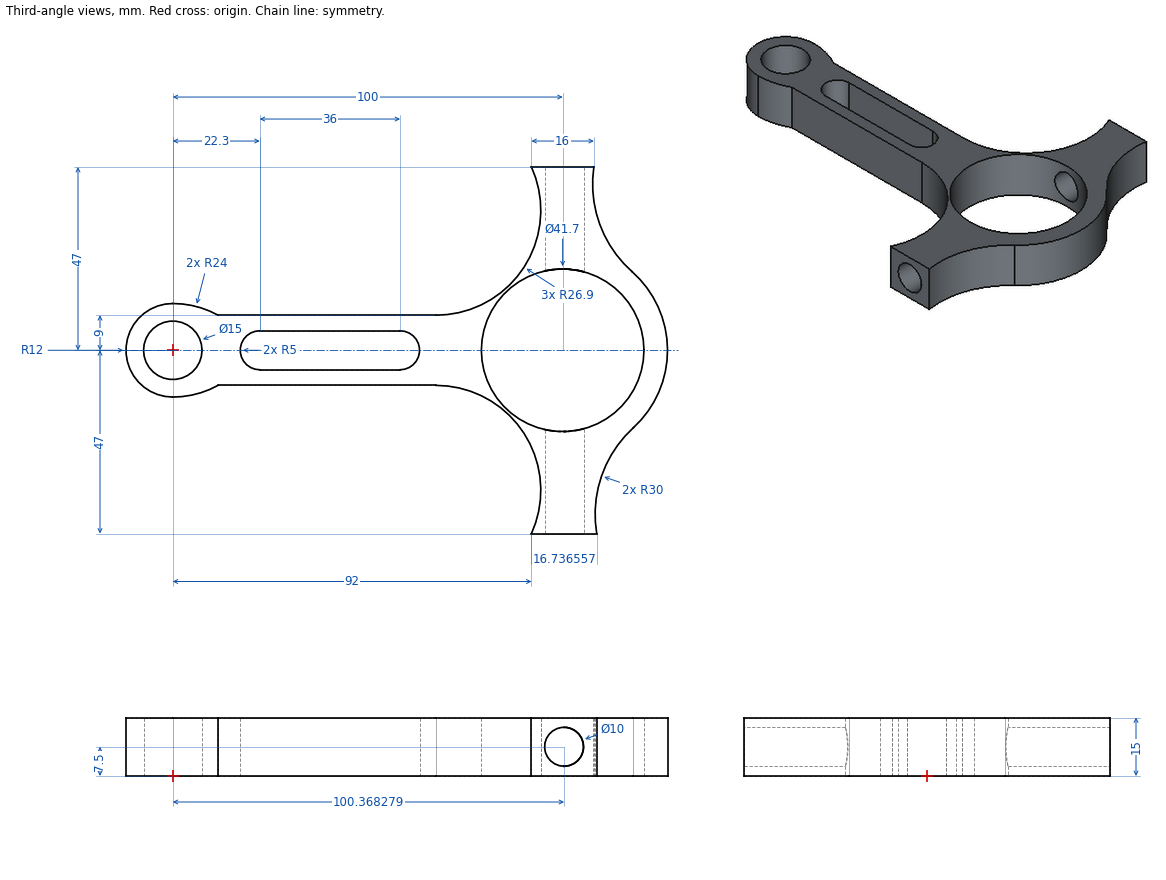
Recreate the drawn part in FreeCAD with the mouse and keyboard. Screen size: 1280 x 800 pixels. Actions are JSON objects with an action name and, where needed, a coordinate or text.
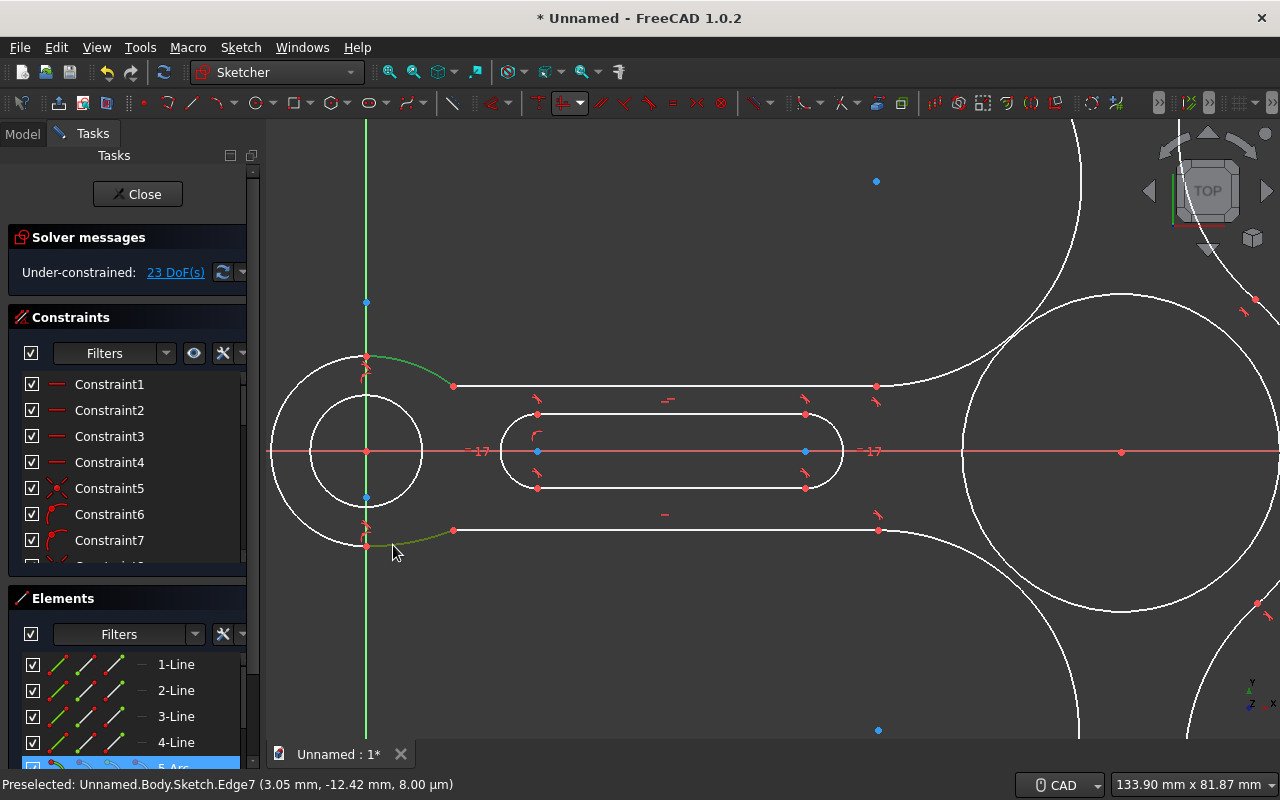
{"action": "left_click", "coordinate": [674, 104]}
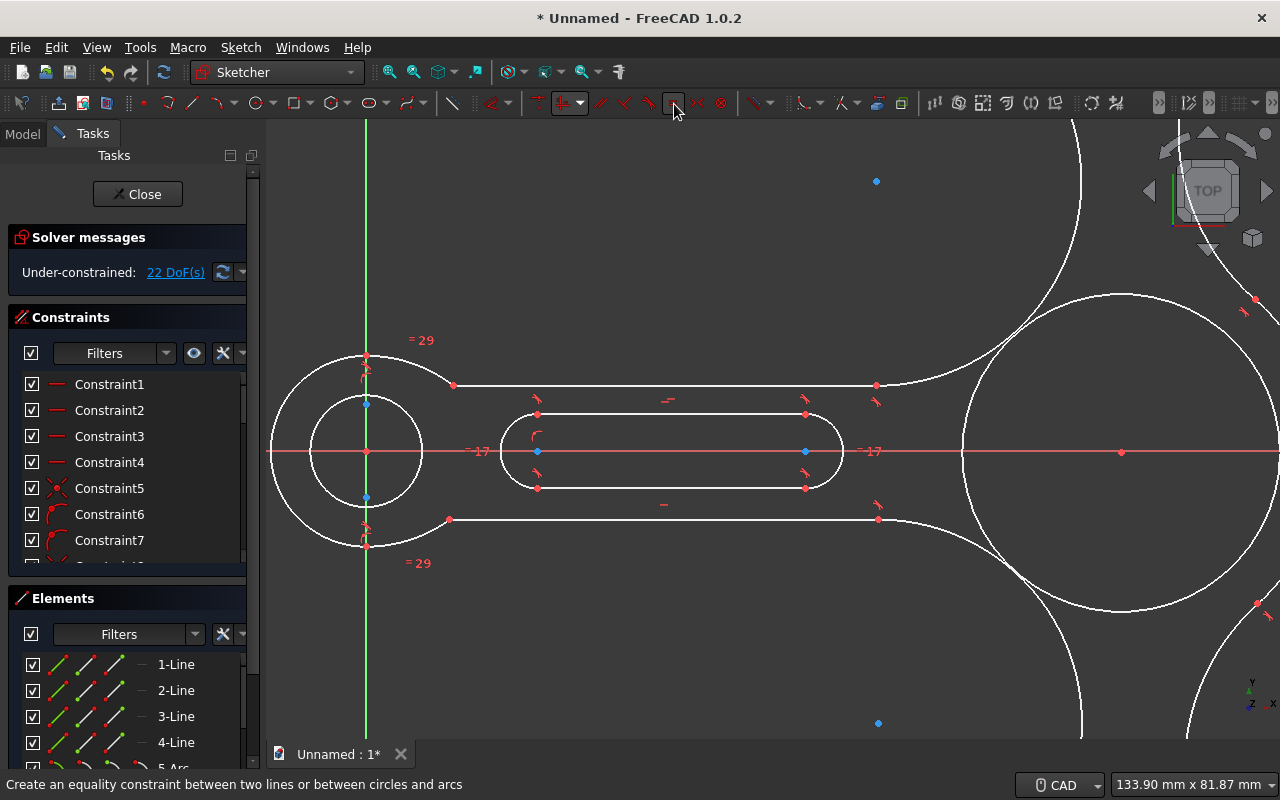
{"action": "left_click", "coordinate": [1079, 689]}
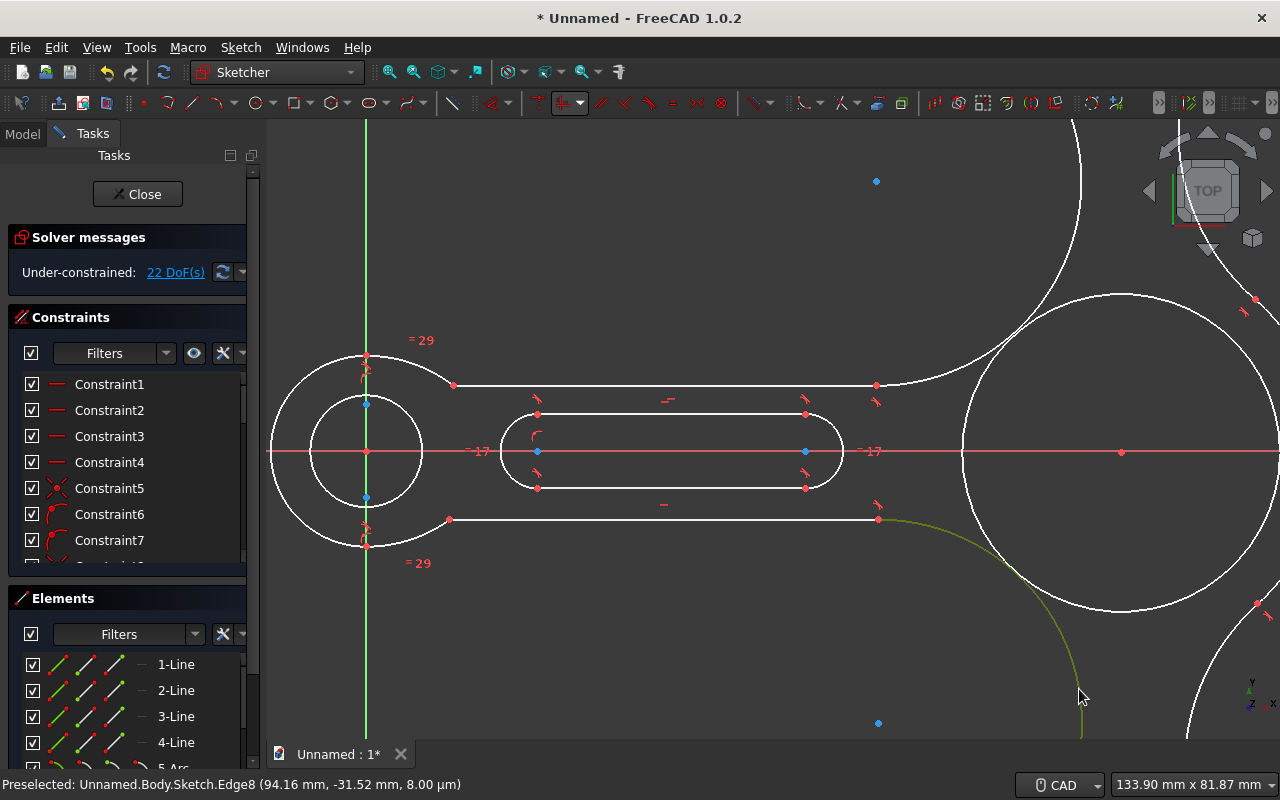
{"action": "scroll", "coordinate": [587, 402], "scroll_direction": "down", "scroll_amount": 3}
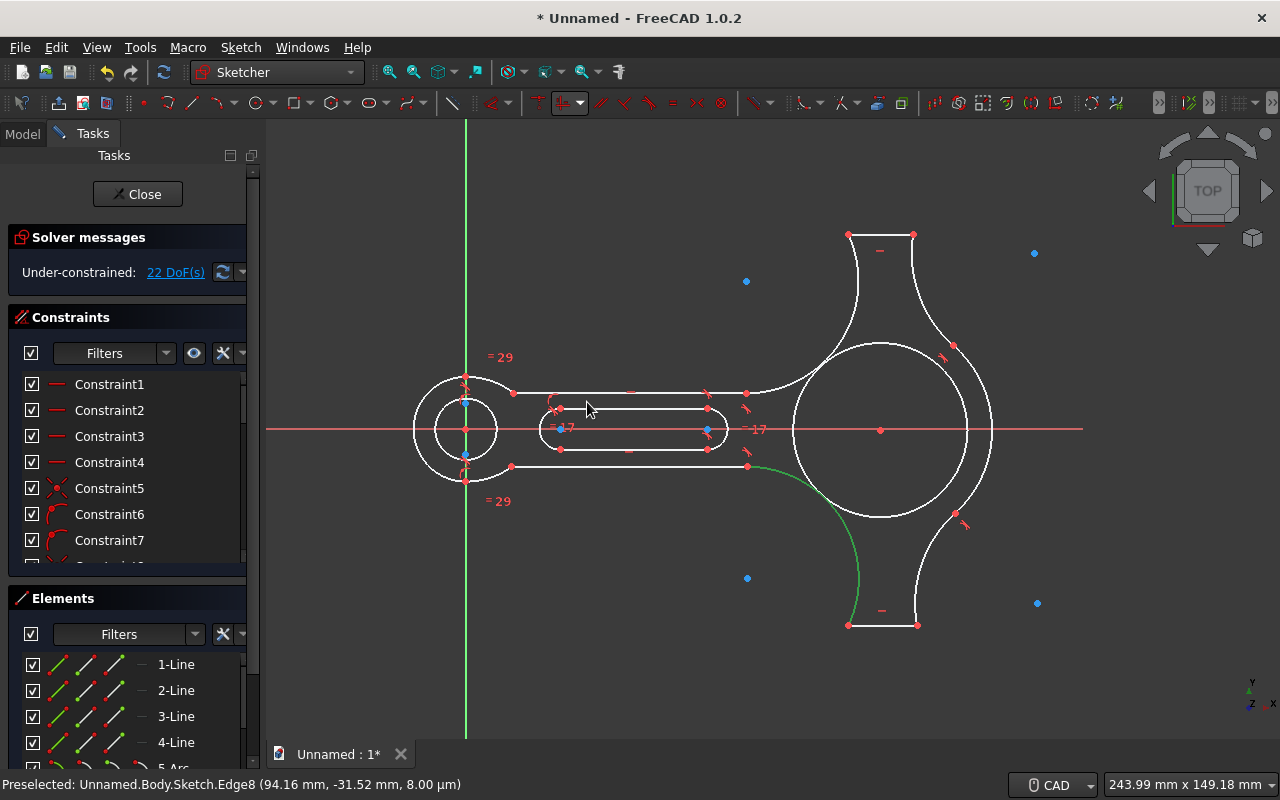
{"action": "left_click", "coordinate": [986, 466]}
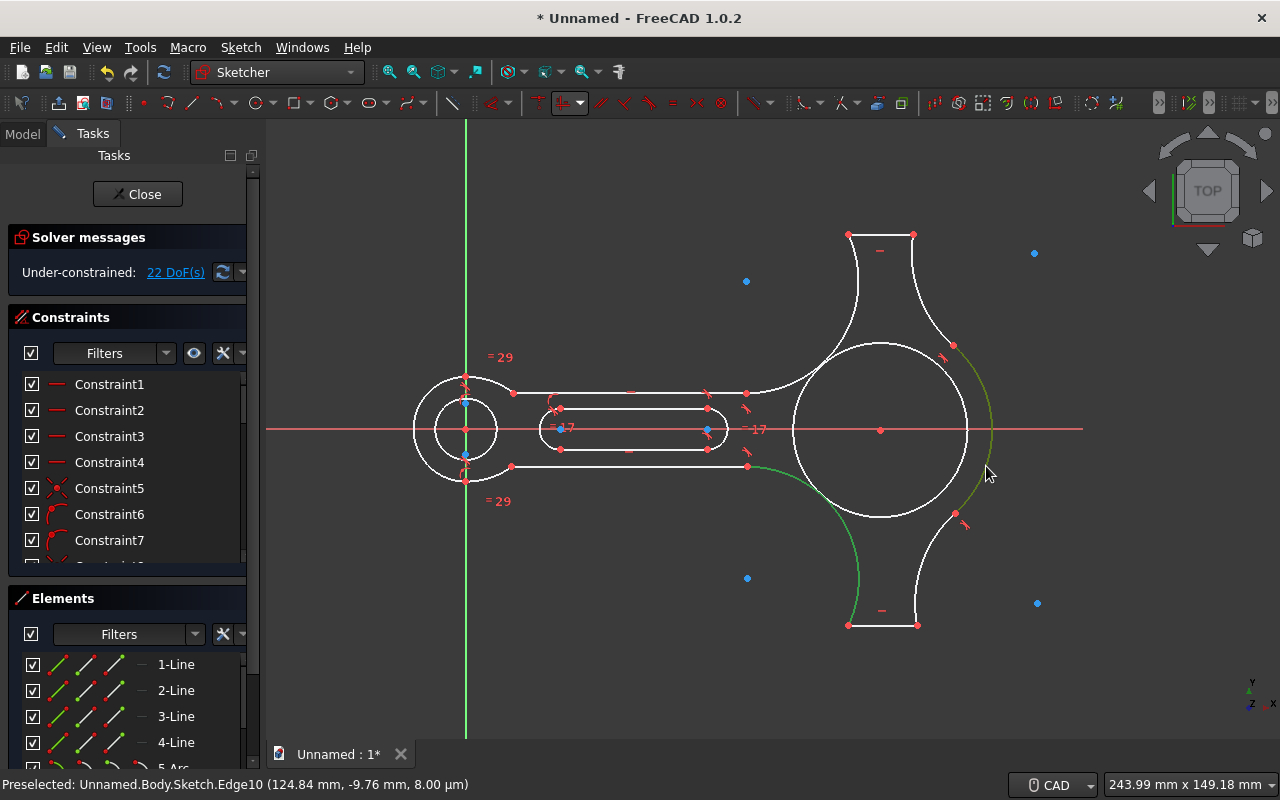
{"action": "left_click", "coordinate": [857, 300]}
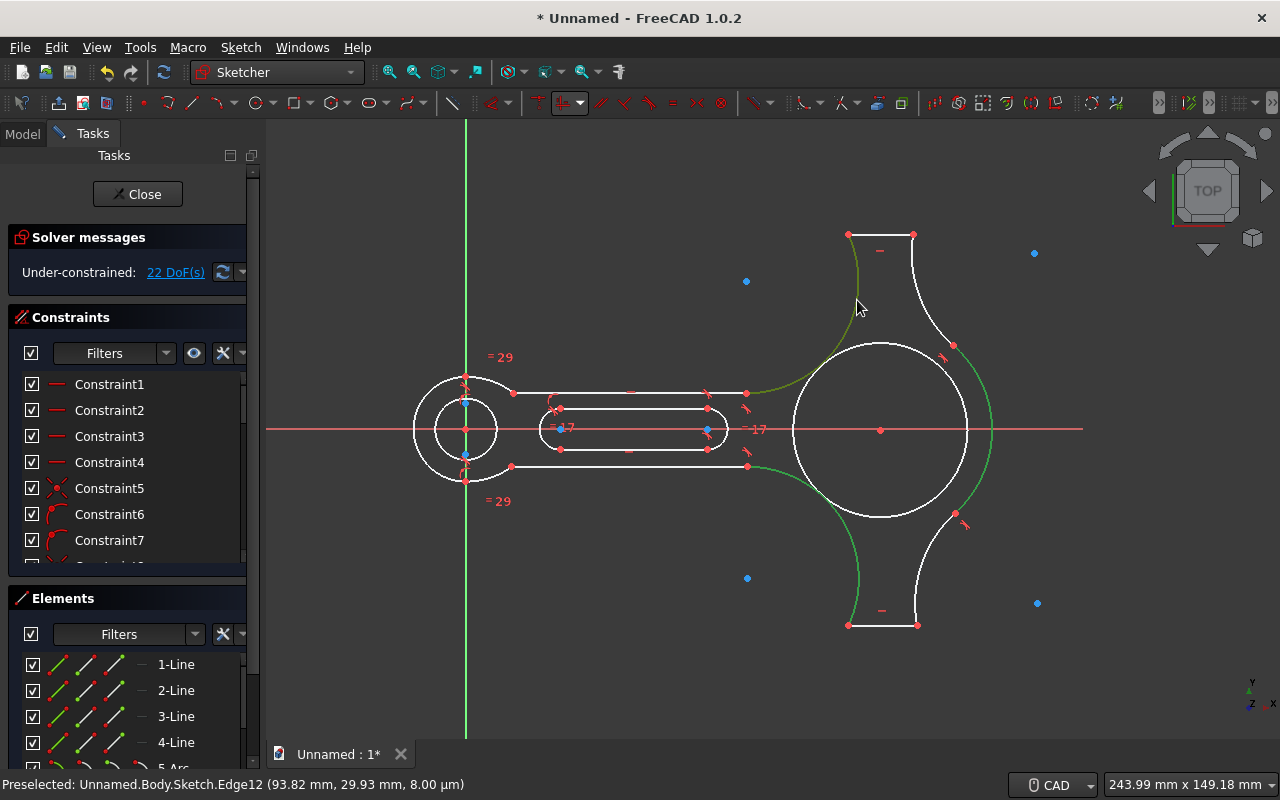
{"action": "left_click", "coordinate": [674, 104]}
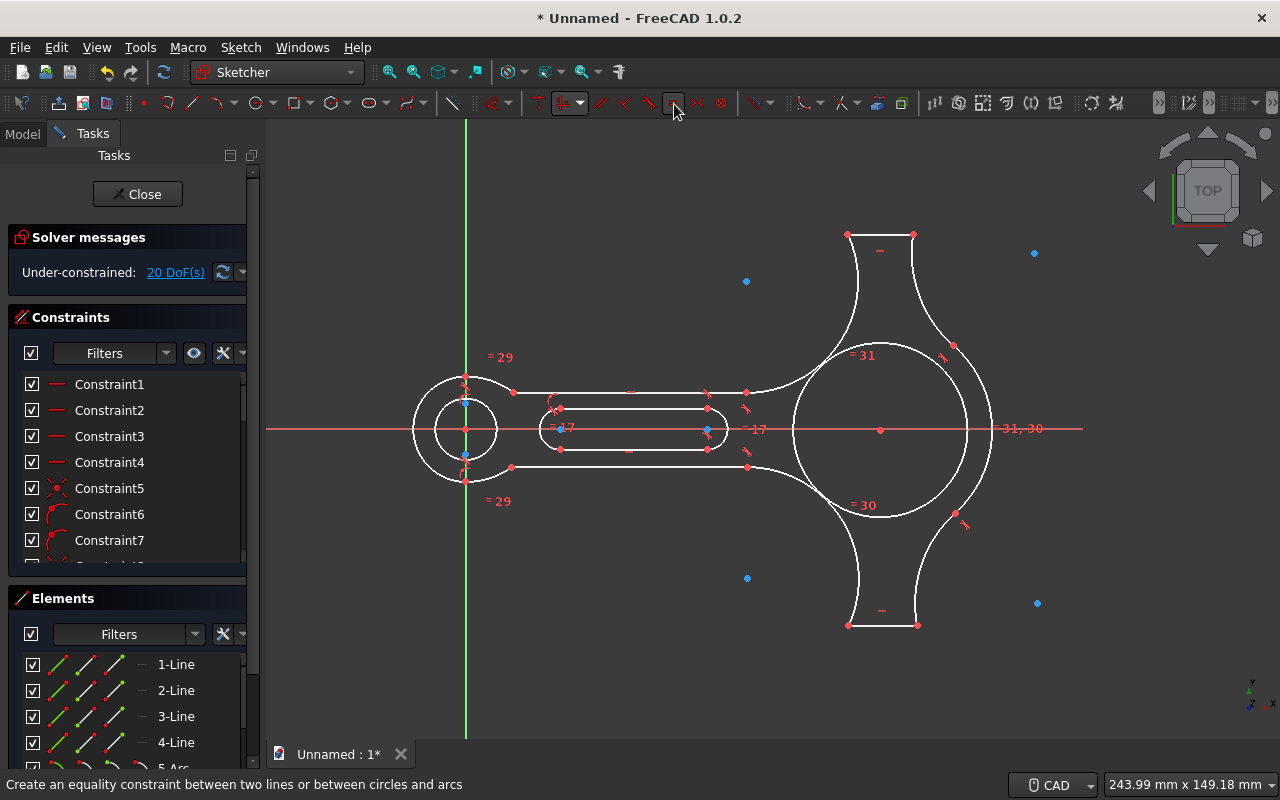
{"action": "left_click", "coordinate": [932, 542]}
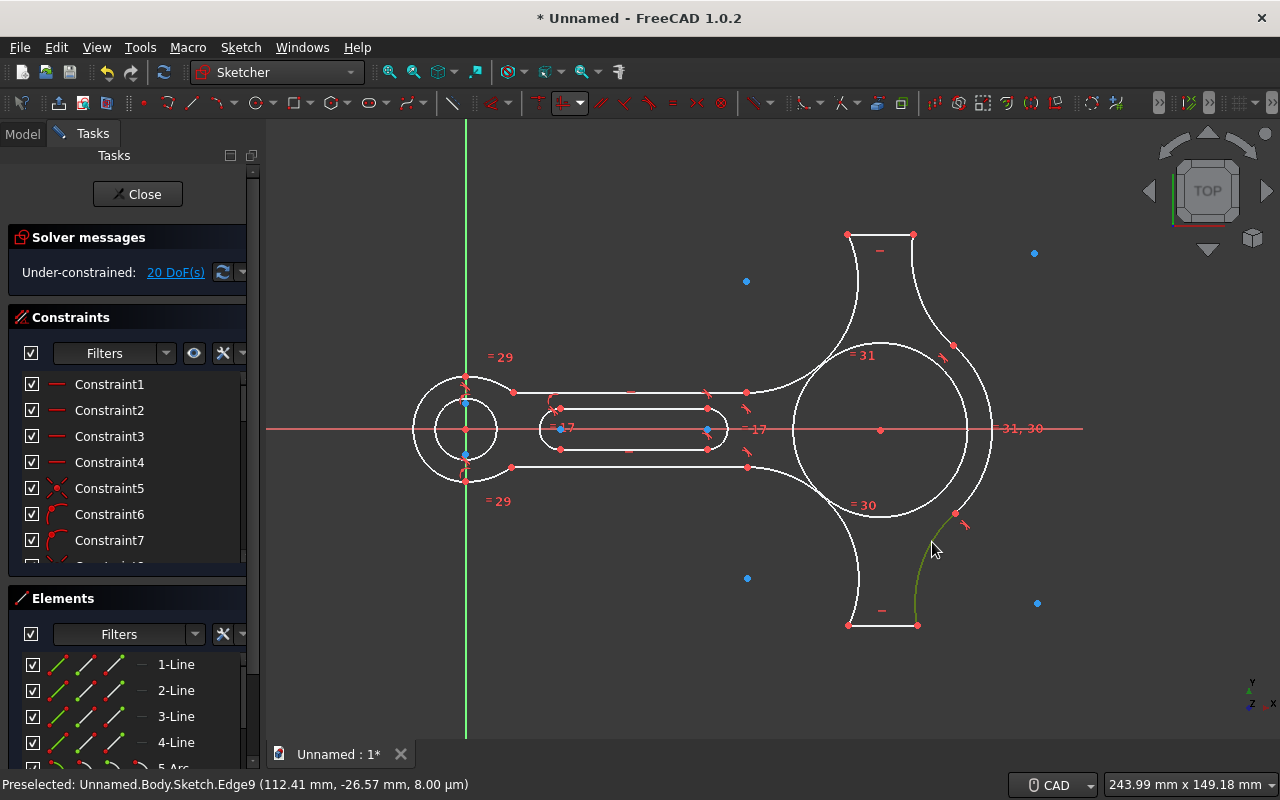
{"action": "left_click", "coordinate": [913, 272]}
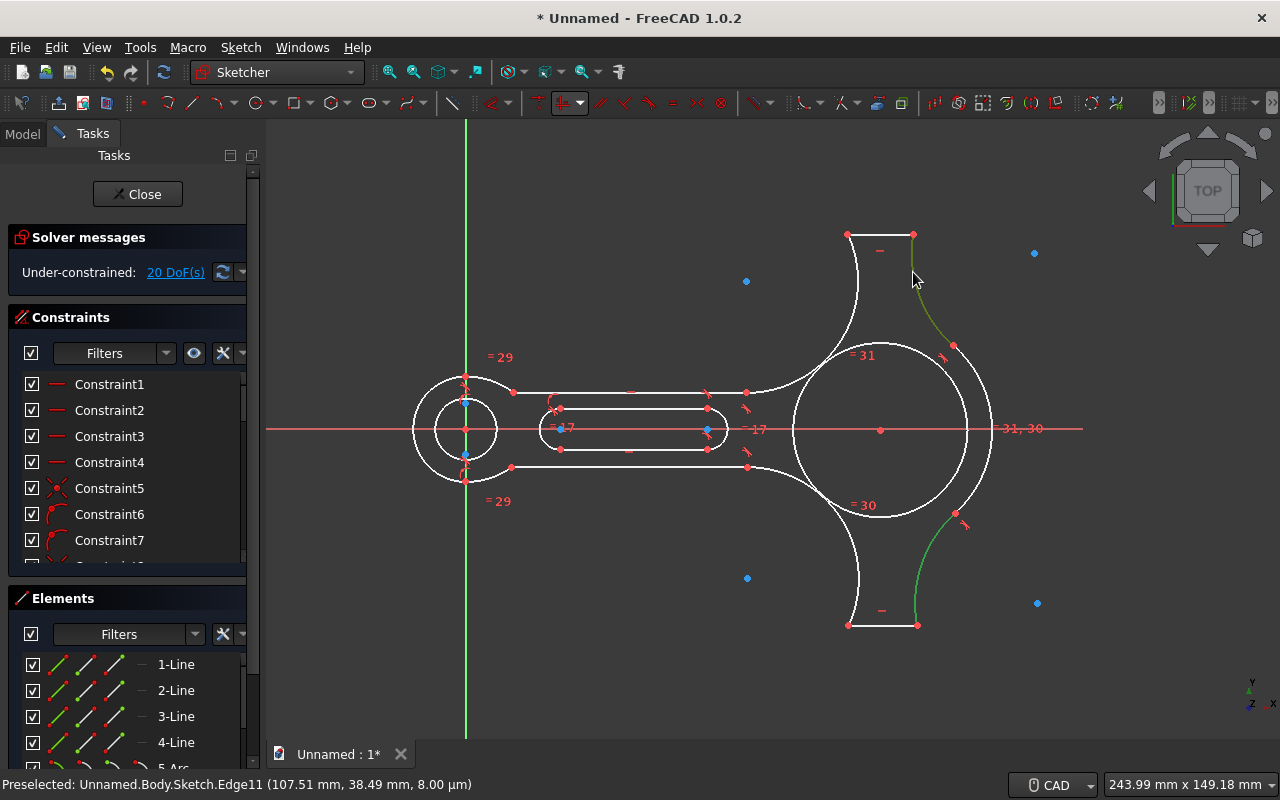
{"action": "left_click", "coordinate": [674, 104]}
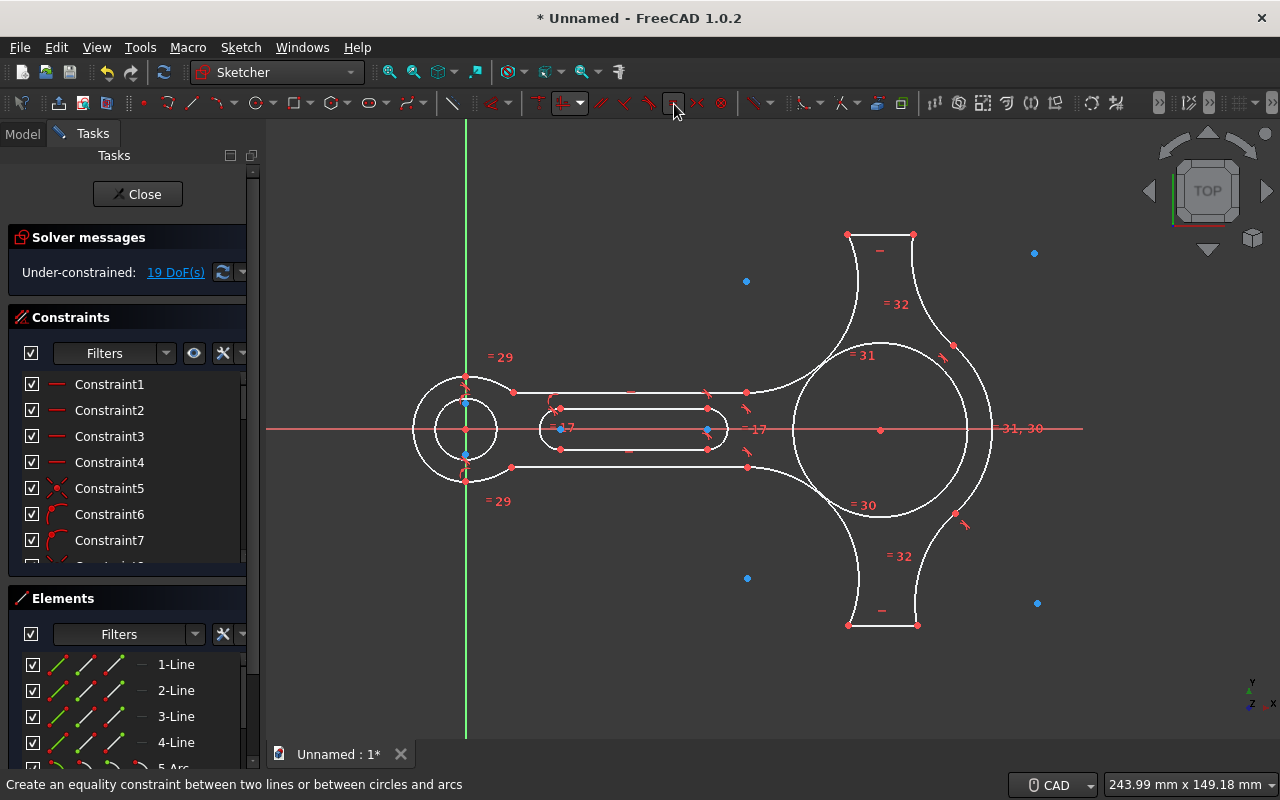
{"action": "left_click", "coordinate": [880, 430]}